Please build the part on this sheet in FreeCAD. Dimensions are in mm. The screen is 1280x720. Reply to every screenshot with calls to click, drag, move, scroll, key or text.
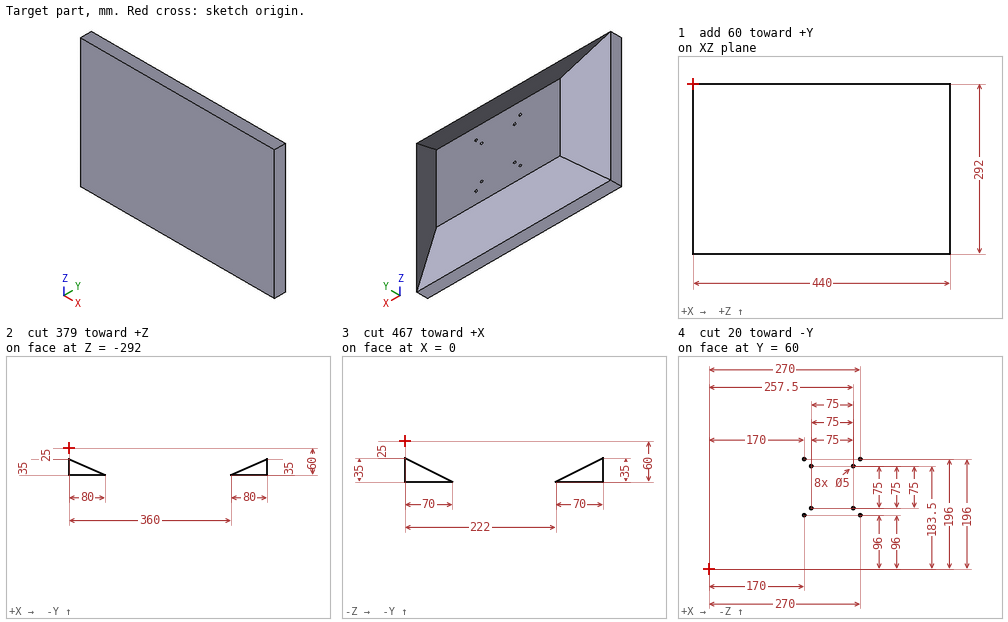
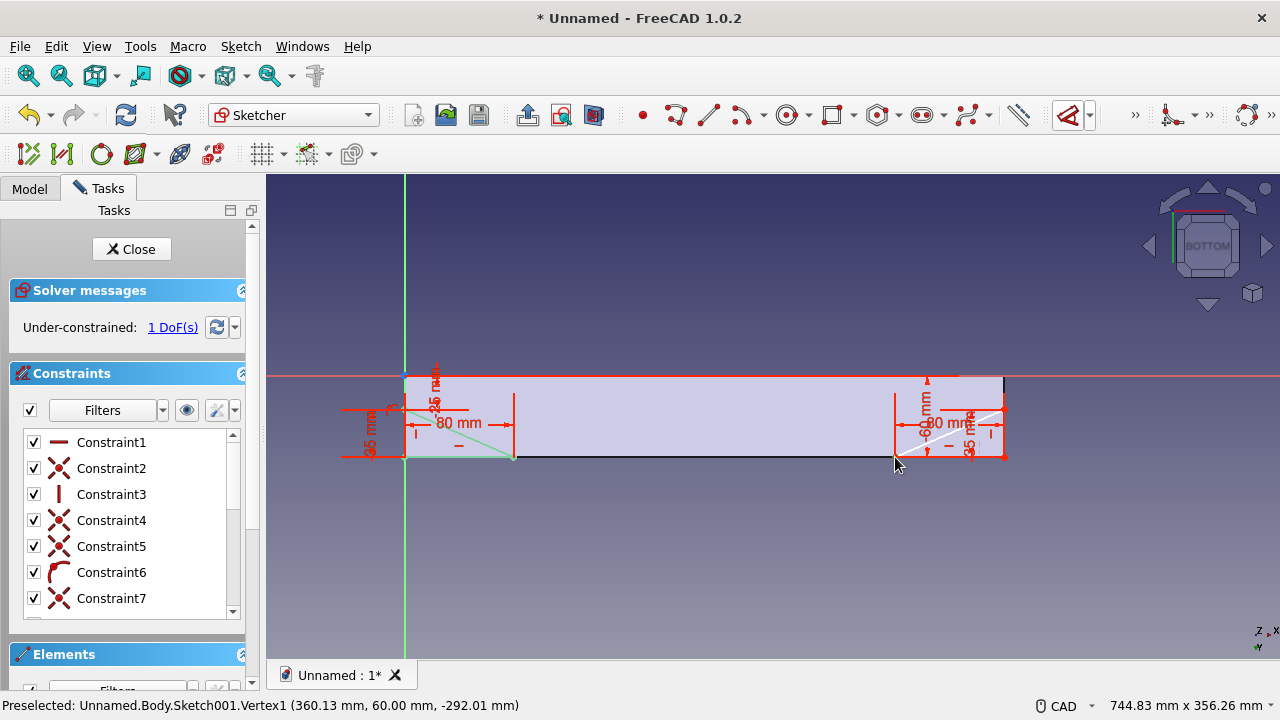
click(1090, 116)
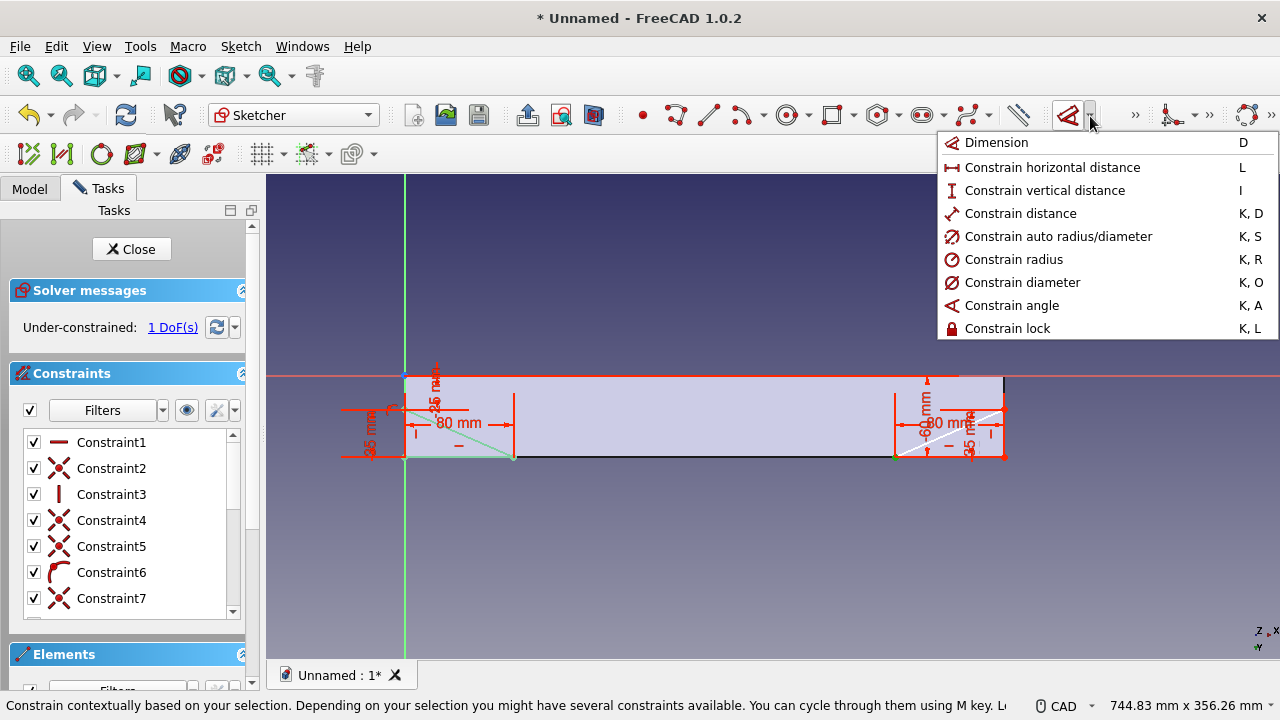
click(1108, 168)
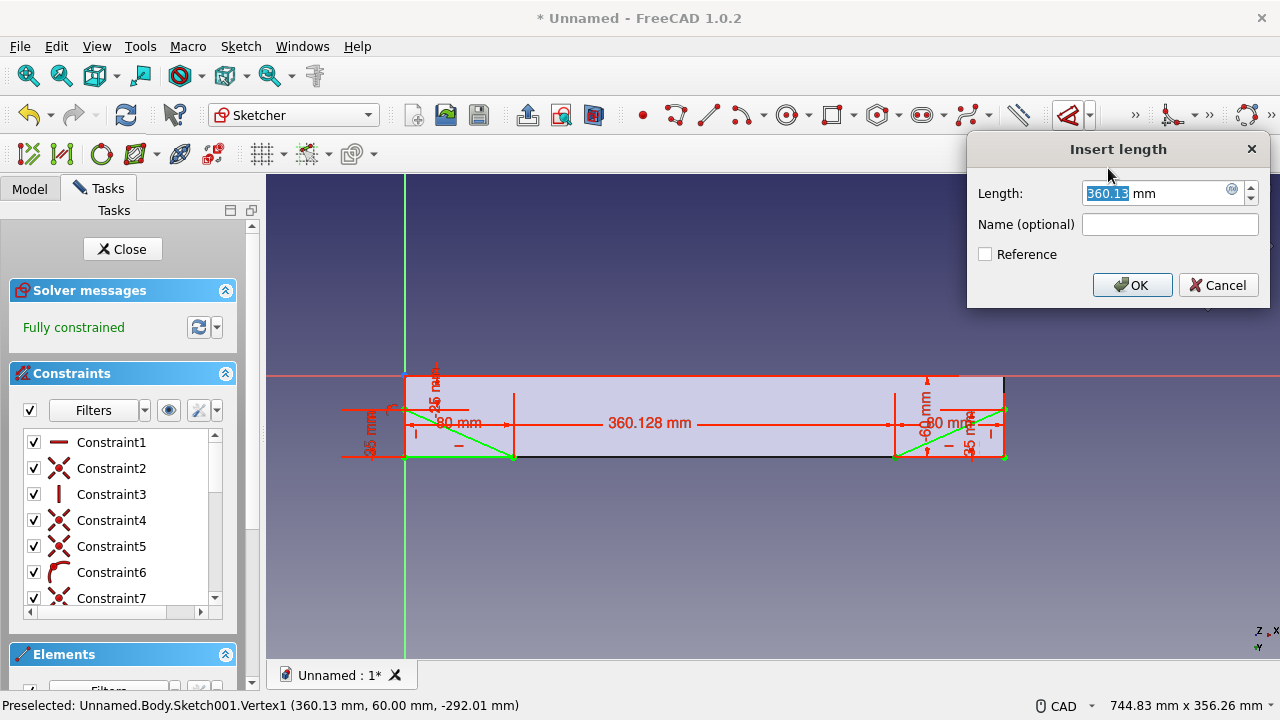
text(360)
key(Return)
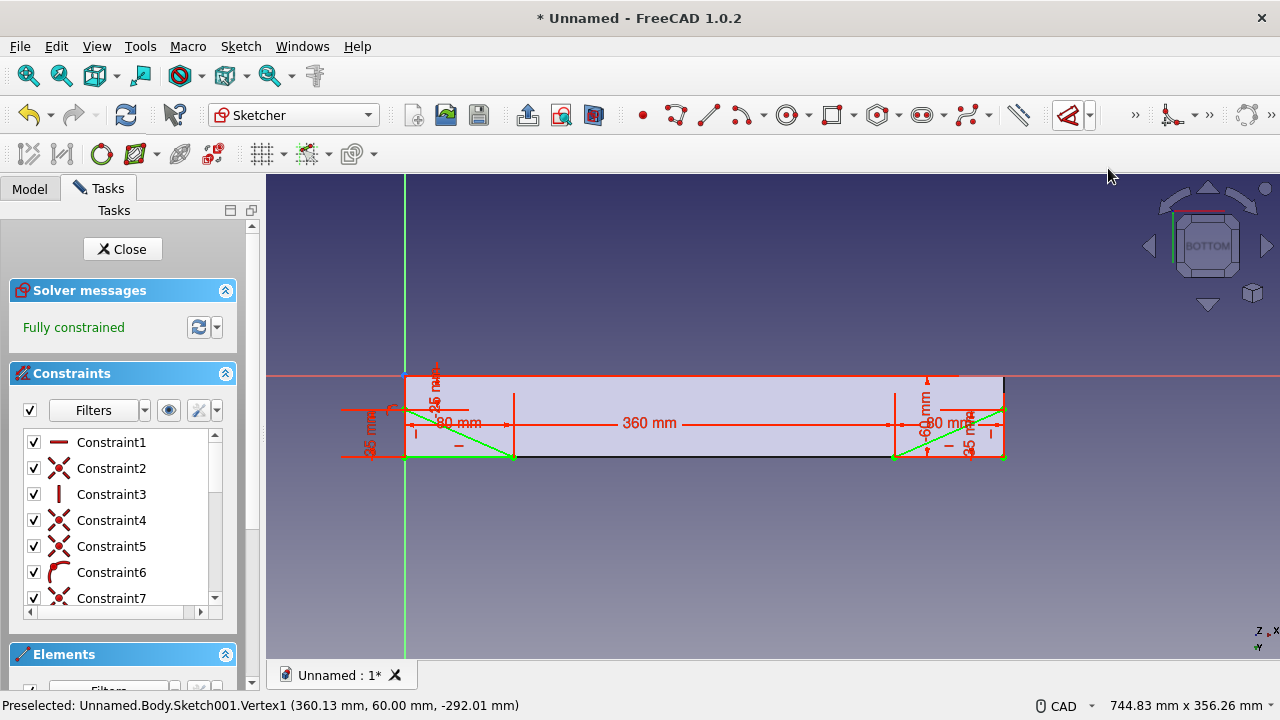
click(123, 249)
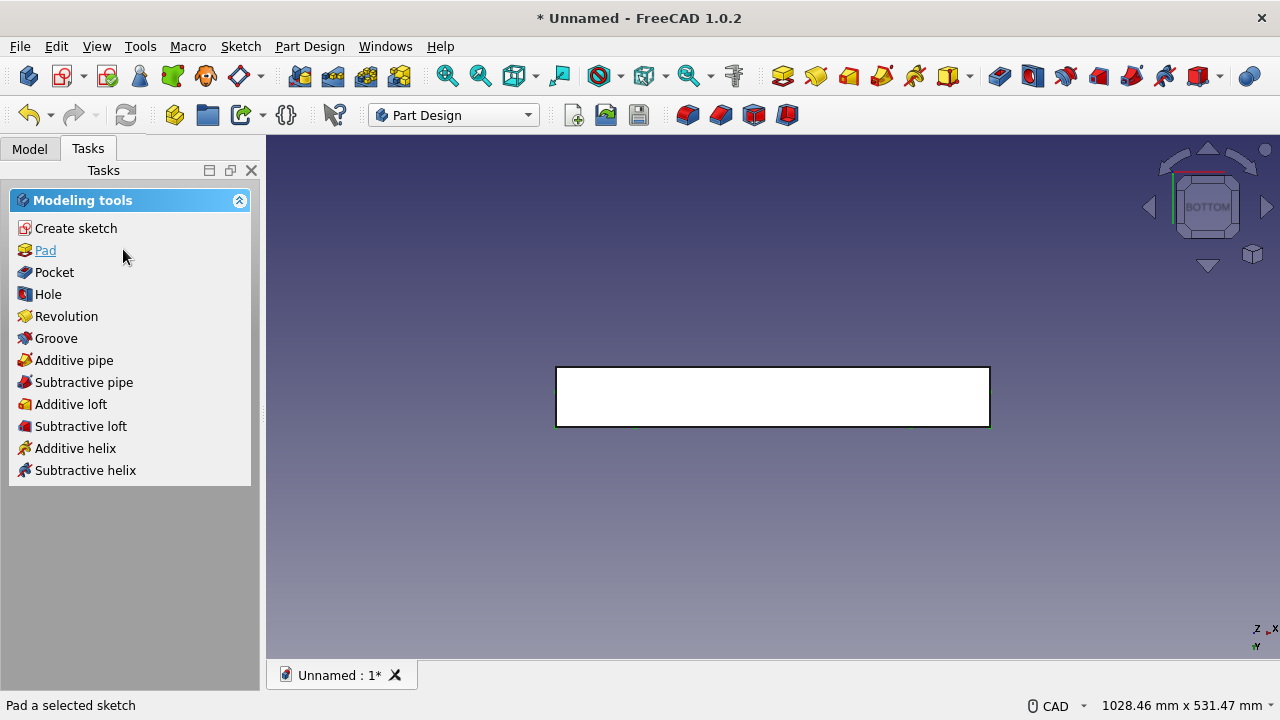
click(1000, 76)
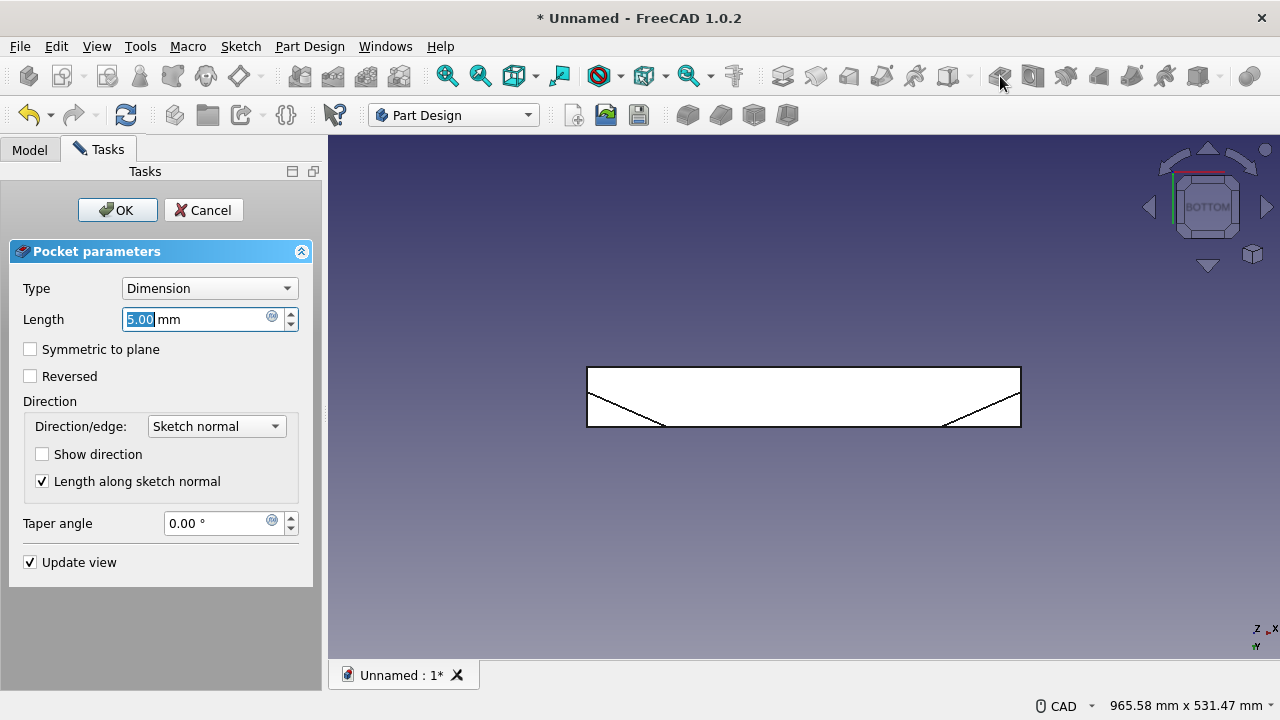
text(379)
key(Tab)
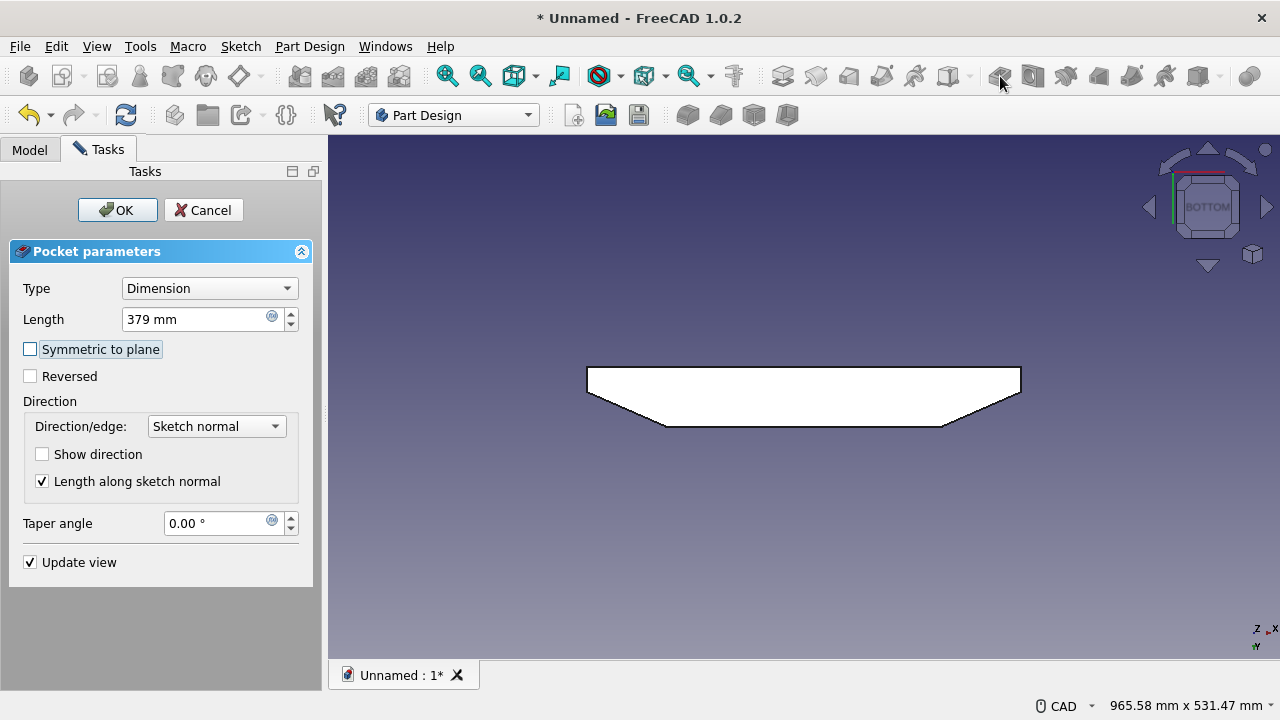
click(118, 210)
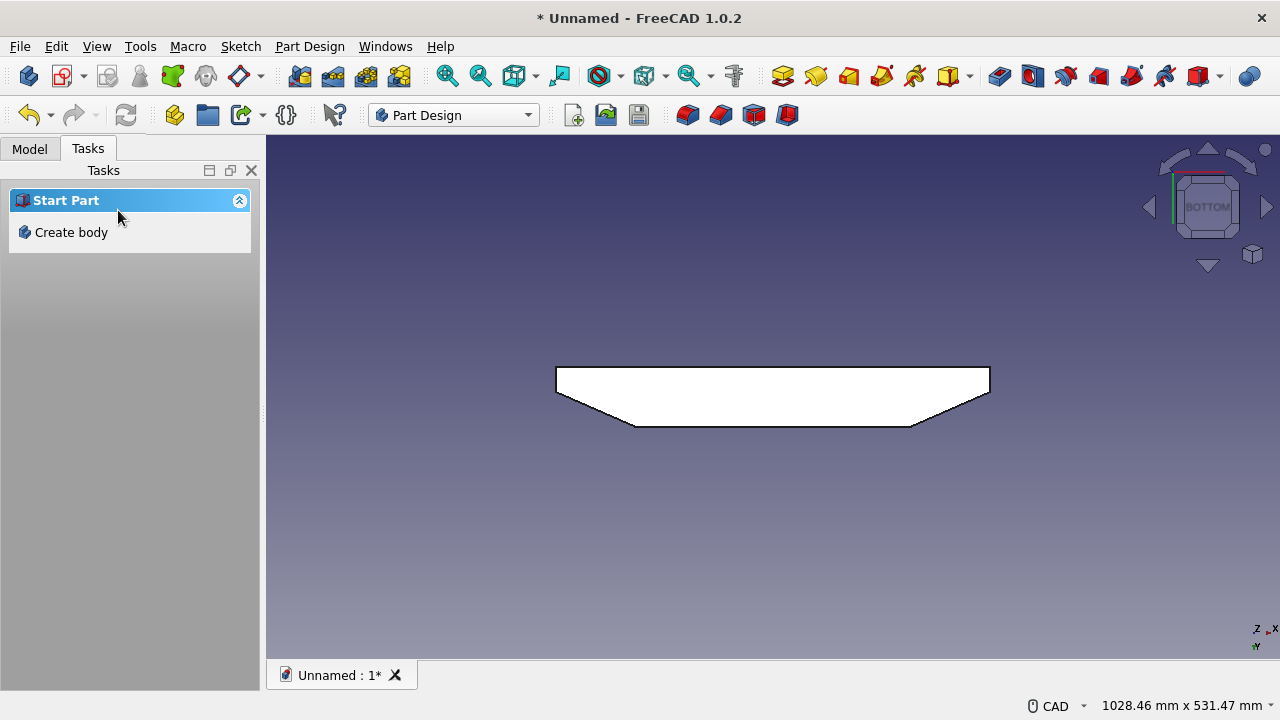
key(v)
key(f)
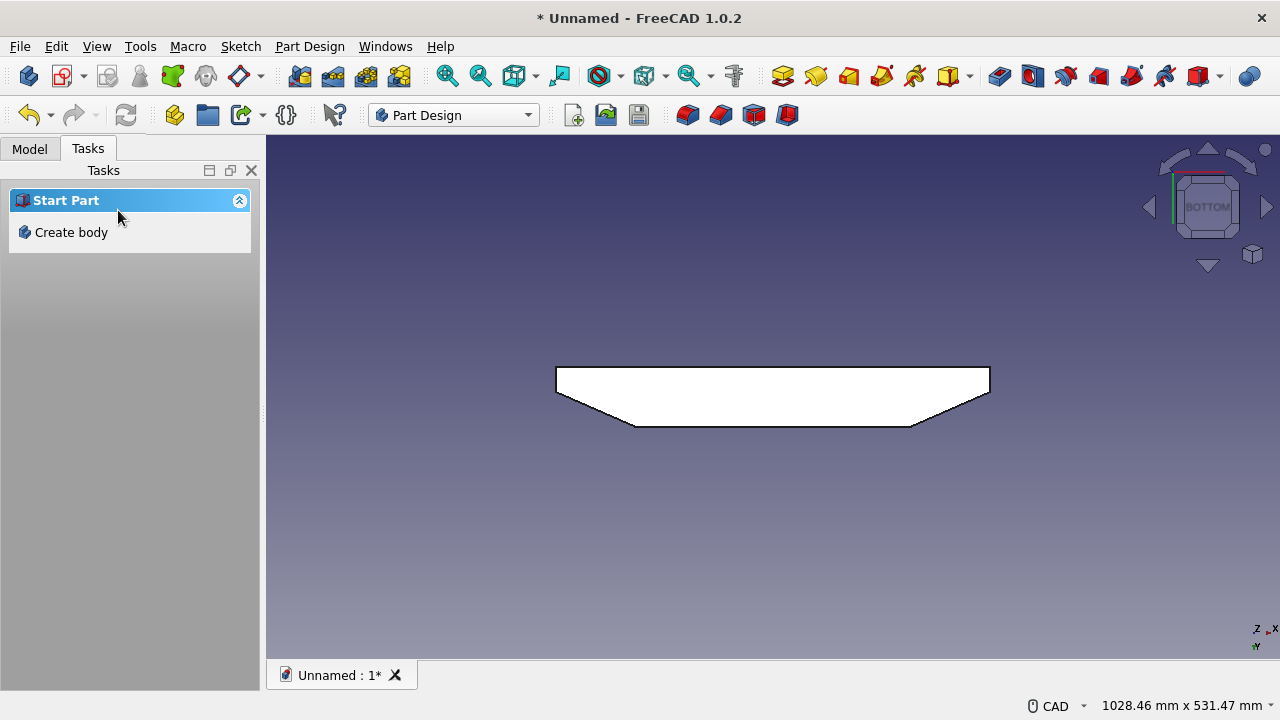
key(6)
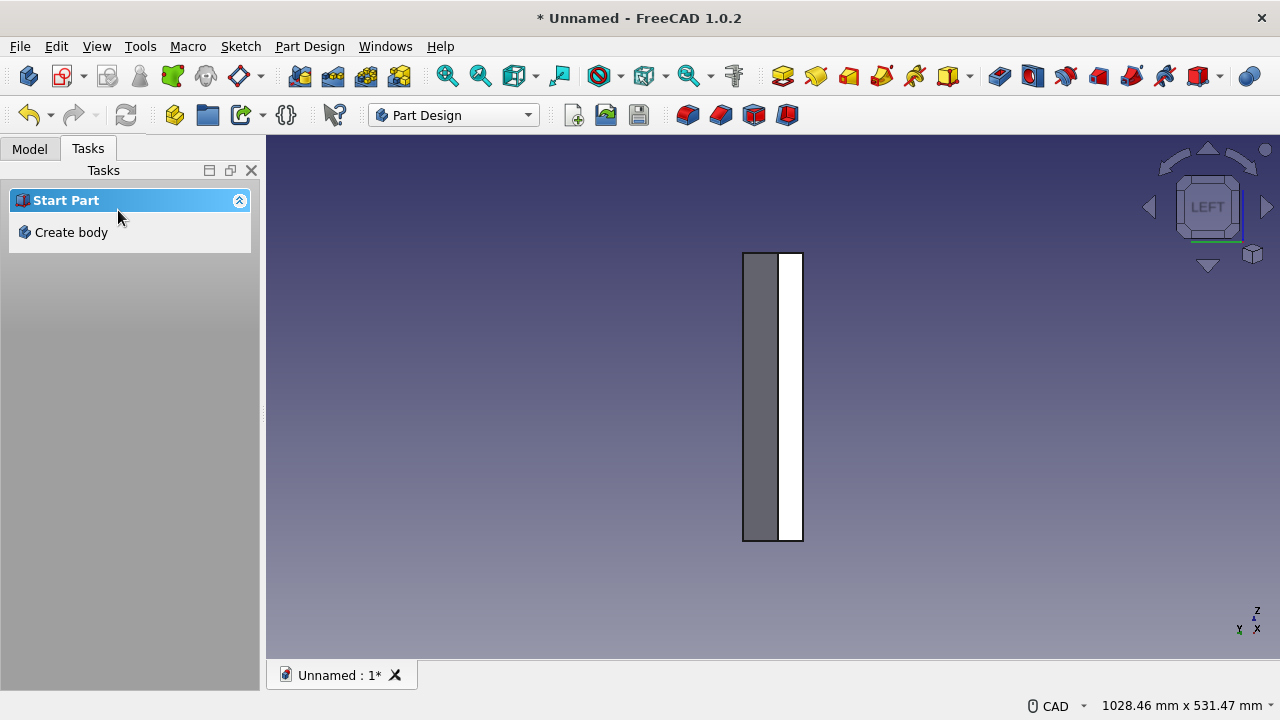
click(790, 519)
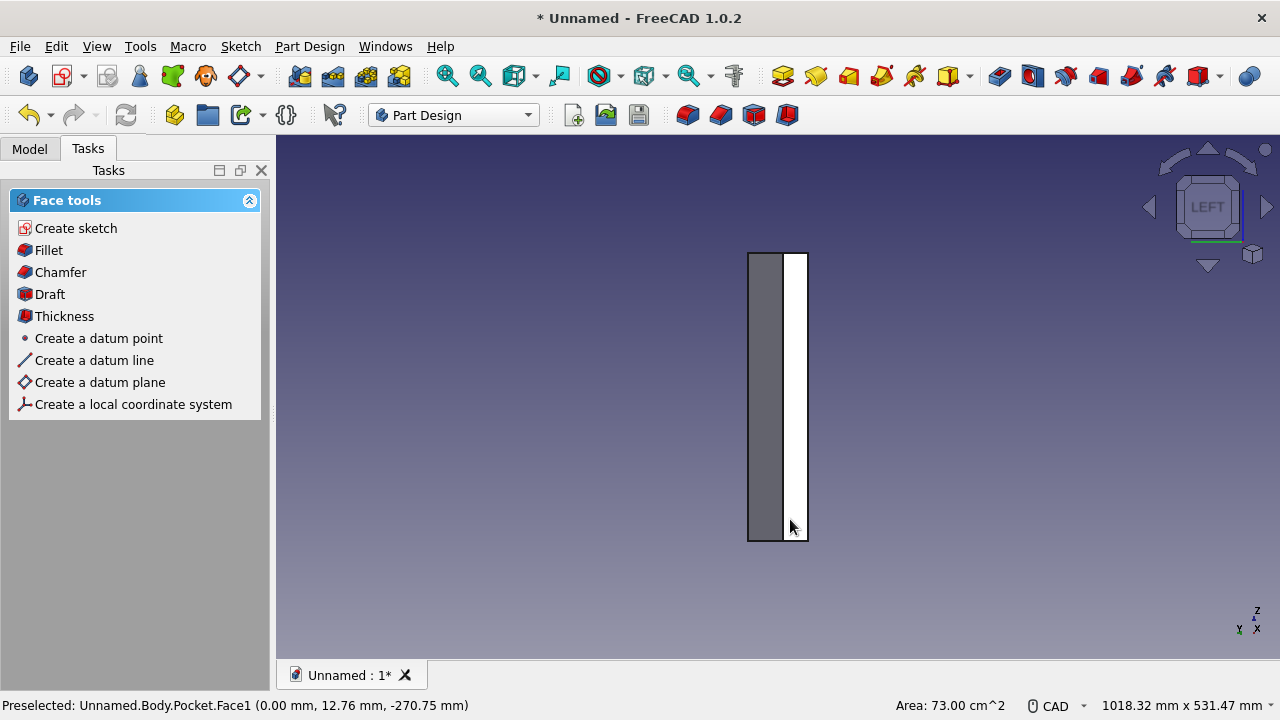
click(62, 76)